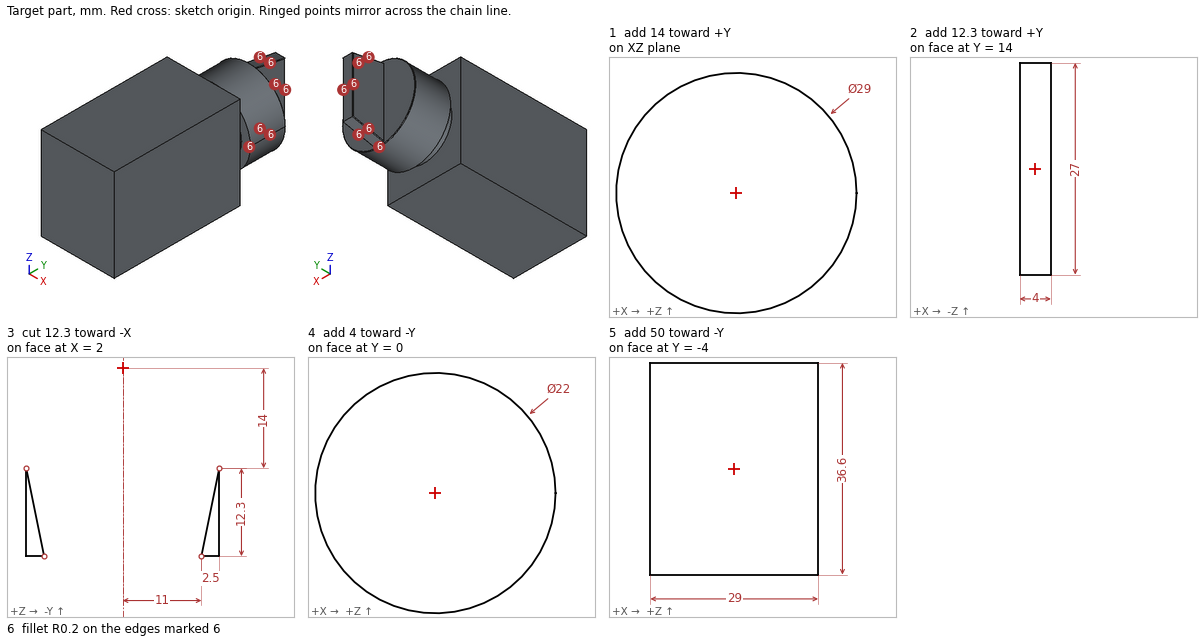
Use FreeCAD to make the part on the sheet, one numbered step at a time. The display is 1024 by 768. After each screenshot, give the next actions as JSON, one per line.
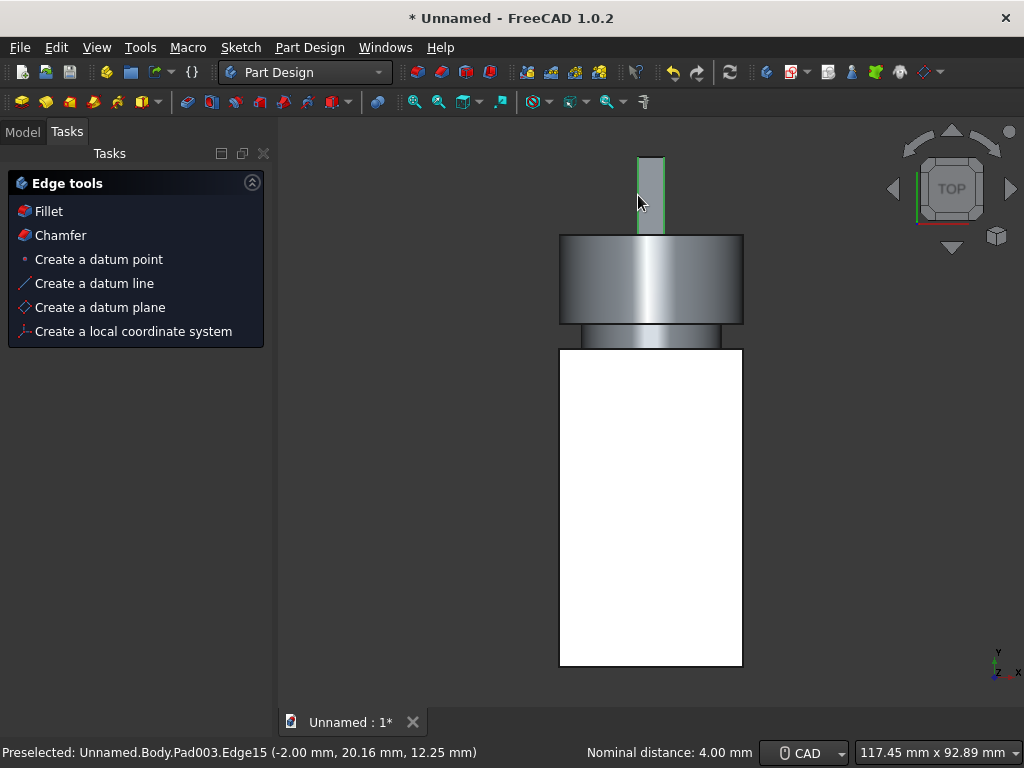
{"action": "key", "text": "0"}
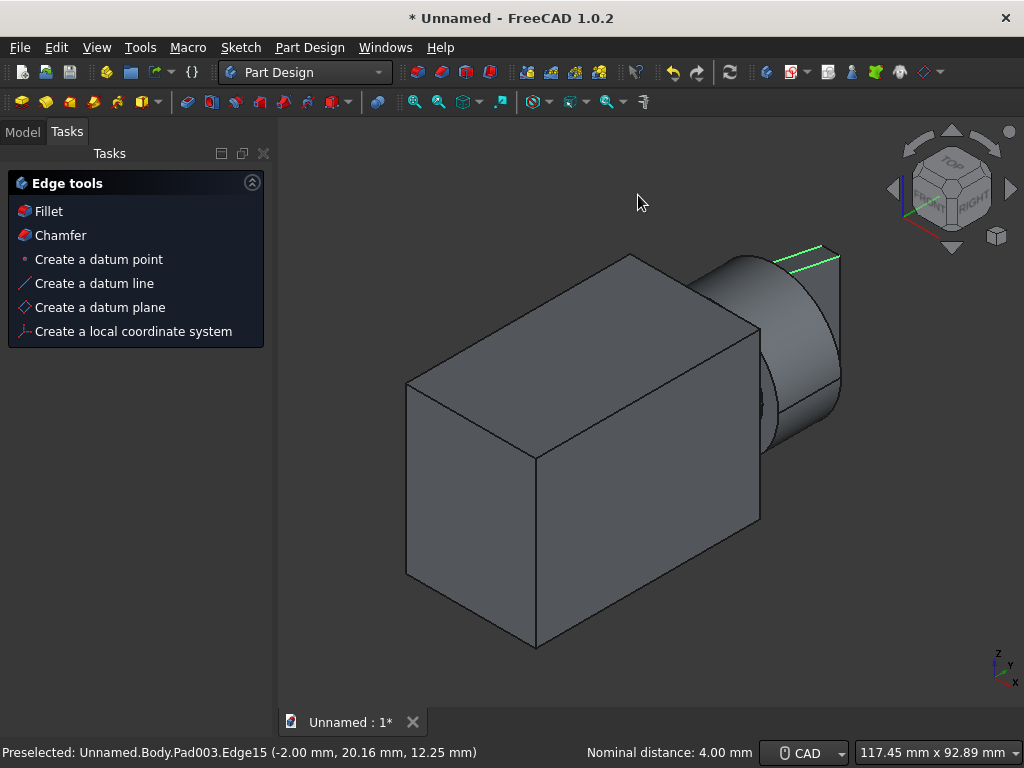
{"action": "key", "text": "1"}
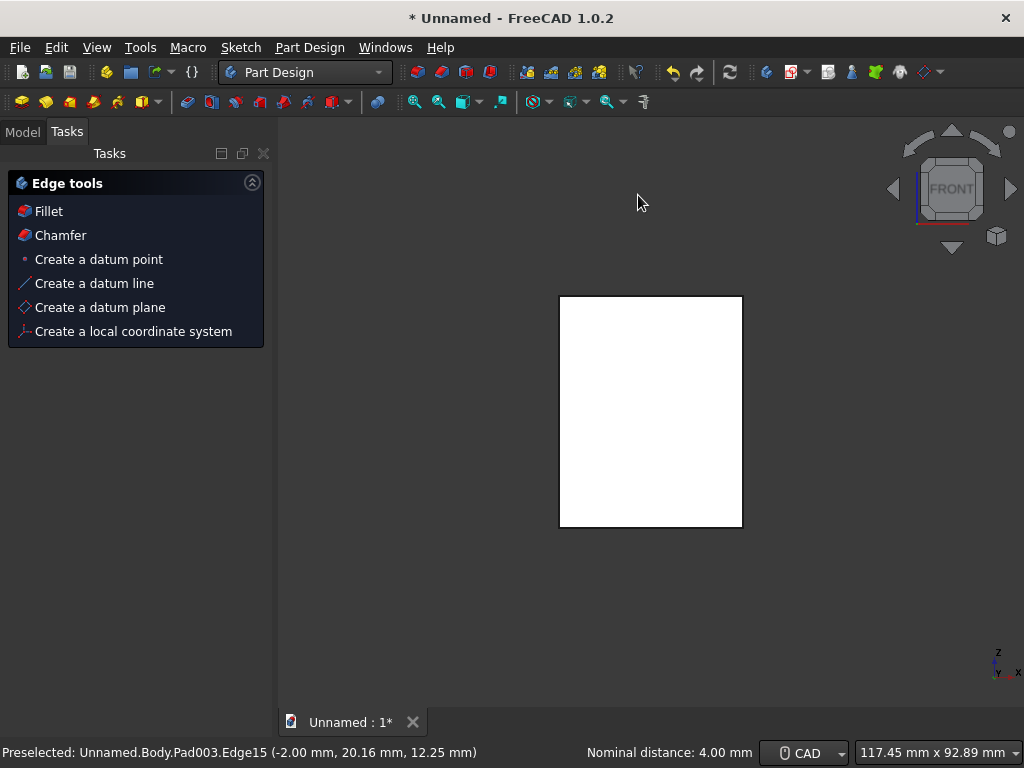
{"action": "key", "text": "v f"}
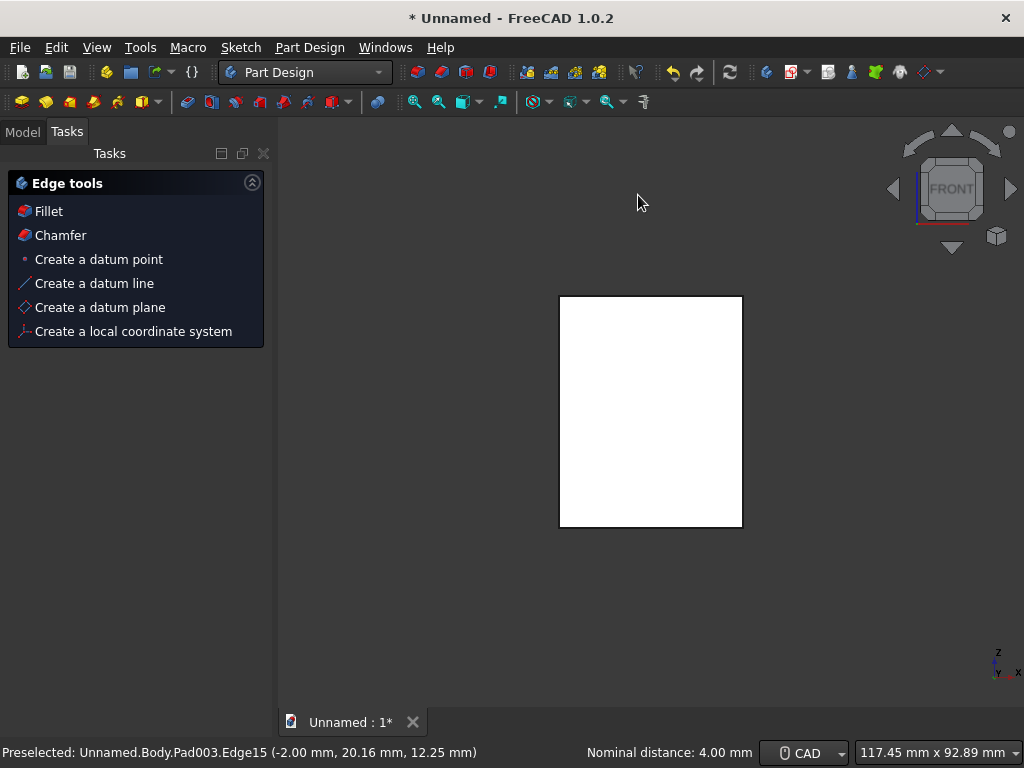
{"action": "key", "text": "3"}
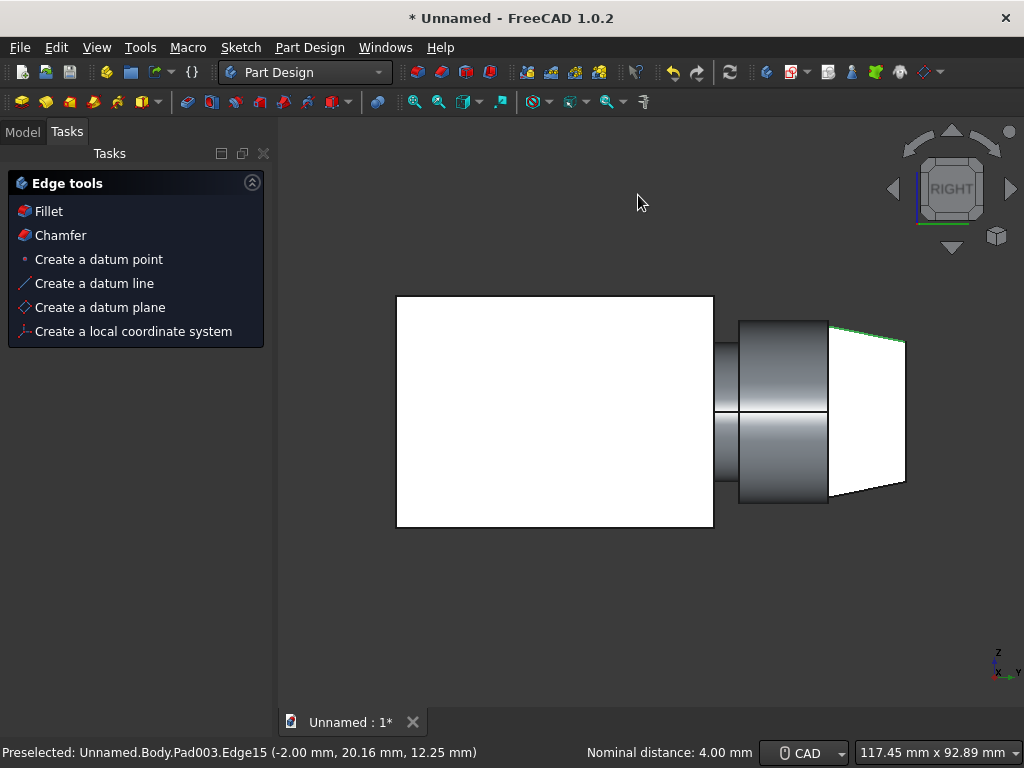
{"action": "left_click", "coordinate": [906, 411], "text": "ctrl"}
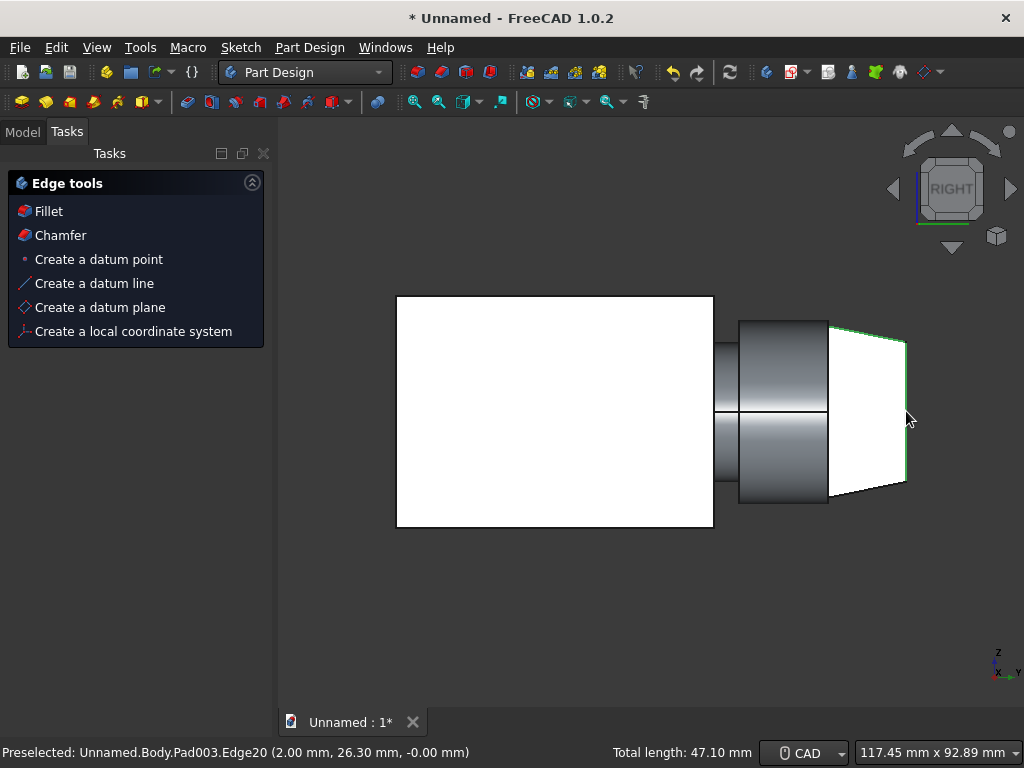
{"action": "left_click", "coordinate": [867, 489], "text": "ctrl"}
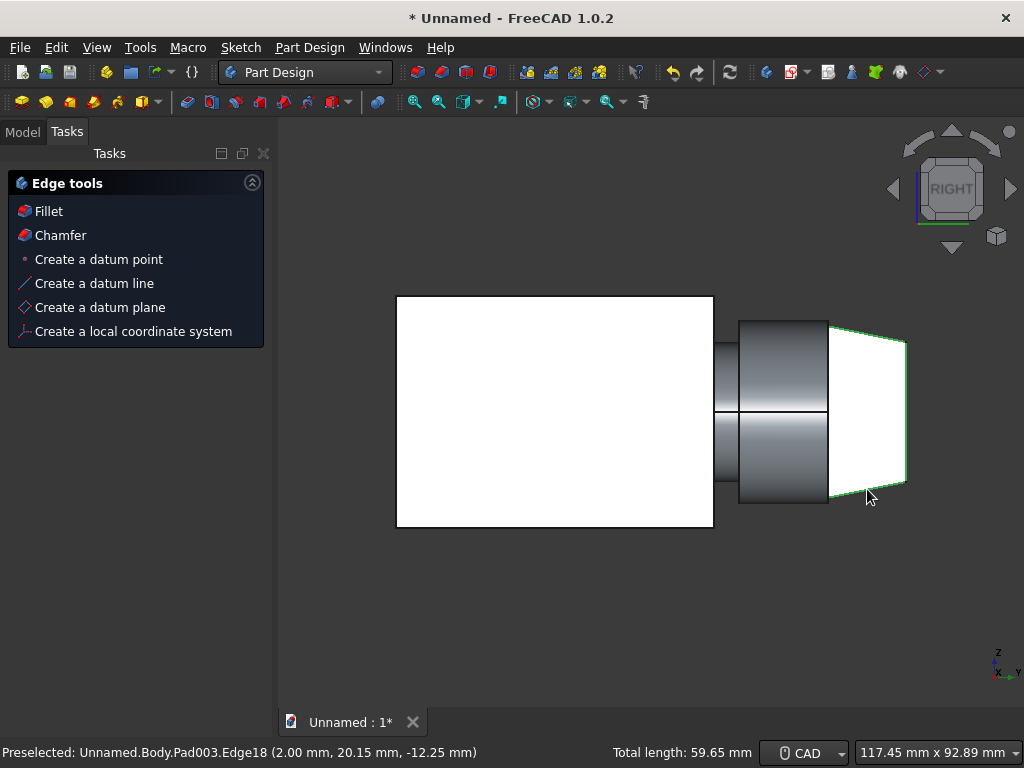
{"action": "left_click", "coordinate": [828, 502], "text": "ctrl"}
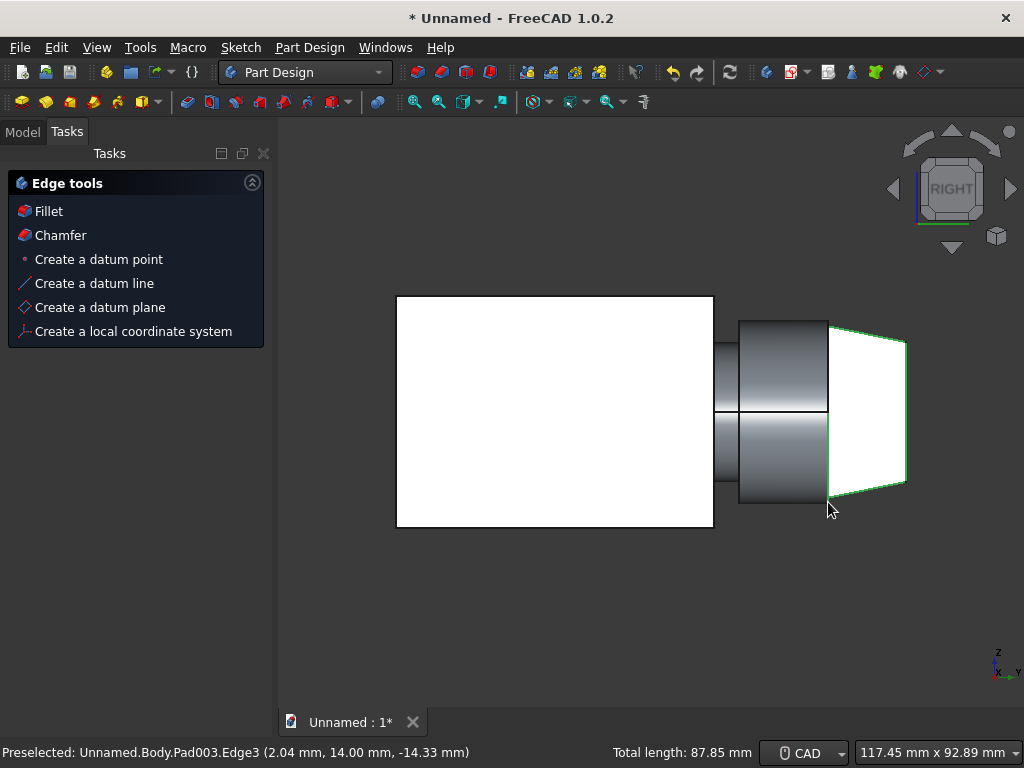
{"action": "key", "text": "5"}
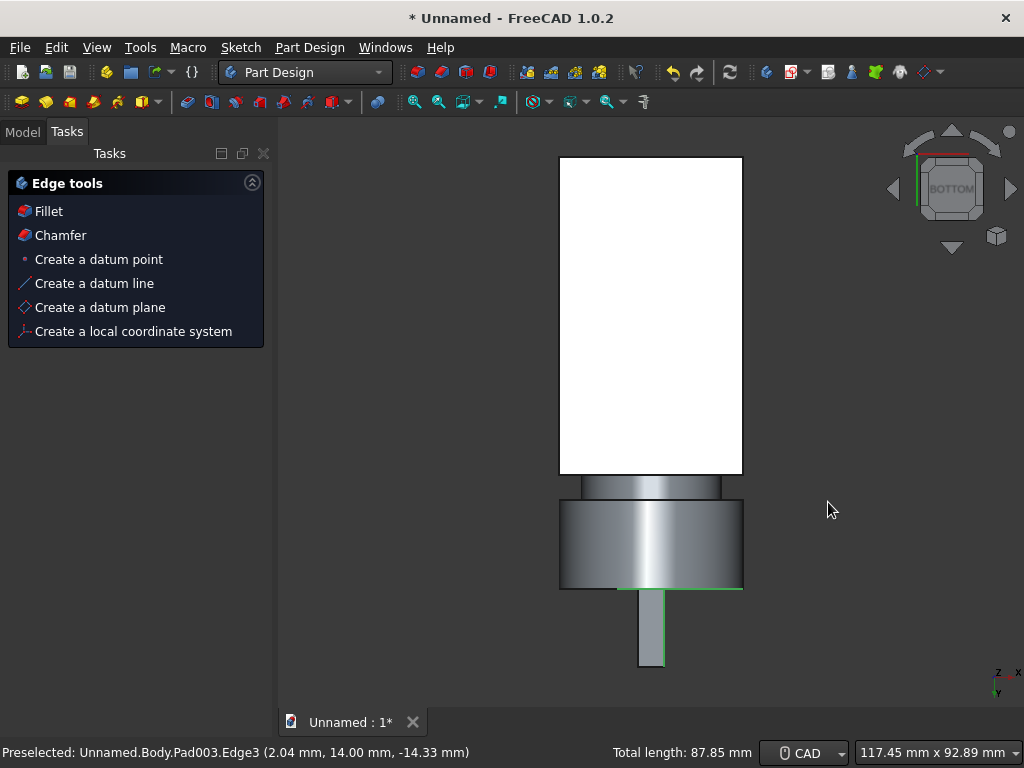
{"action": "left_click", "coordinate": [638, 627], "text": "ctrl"}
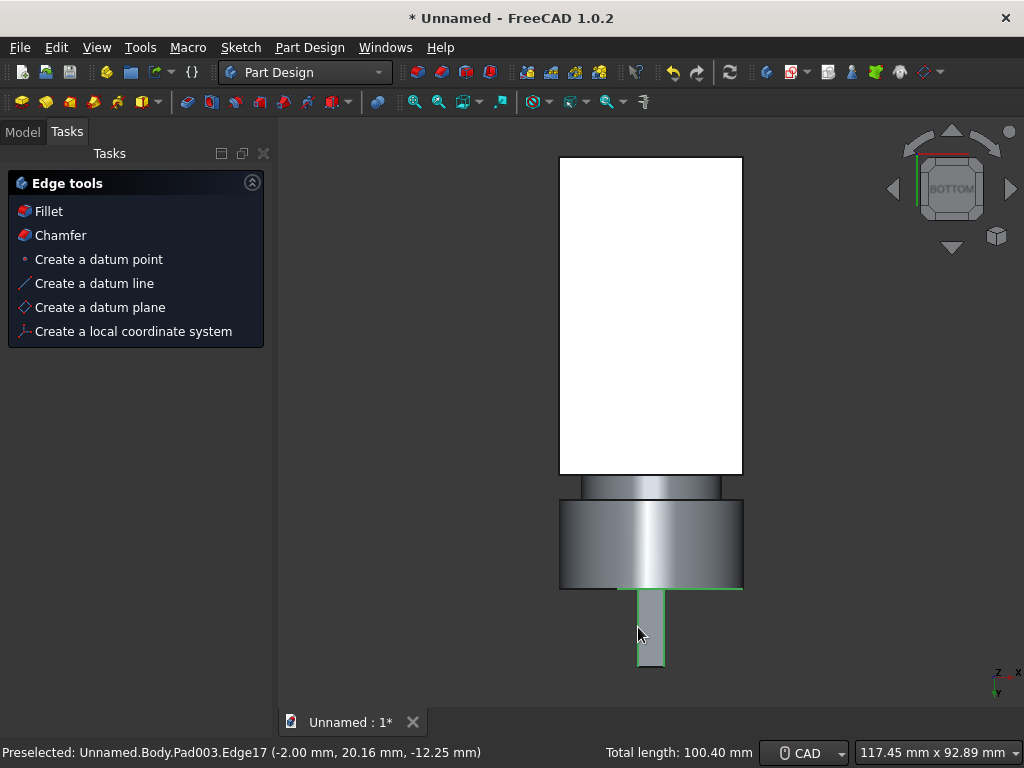
{"action": "key", "text": "4"}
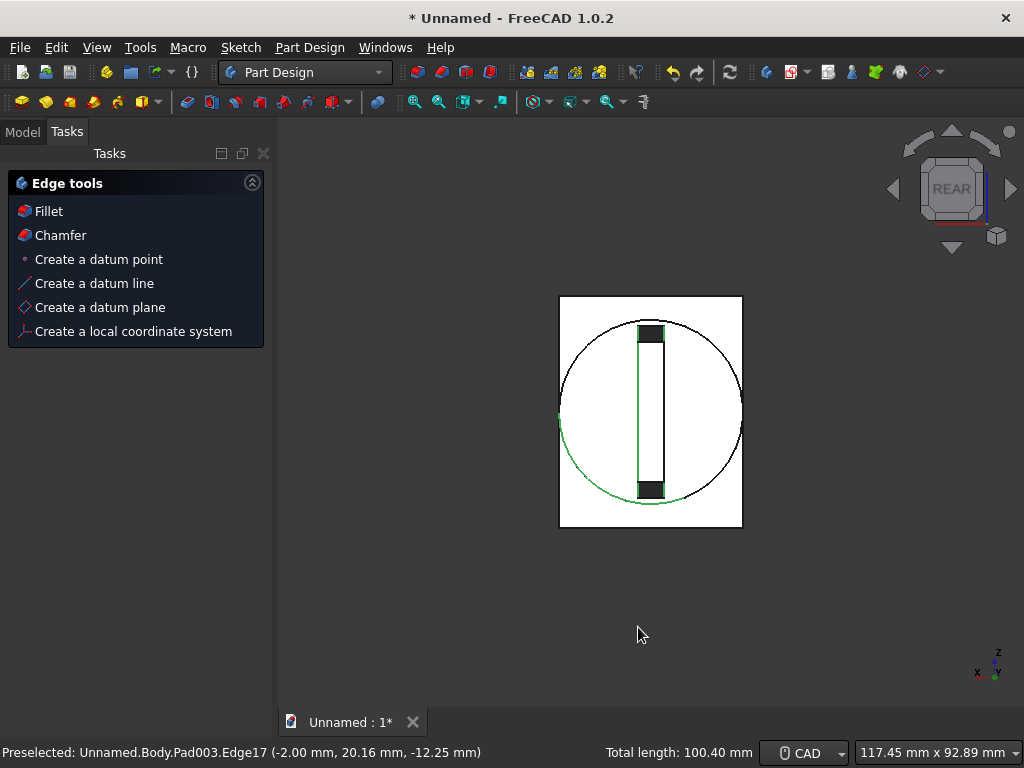
{"action": "left_click", "coordinate": [416, 102]}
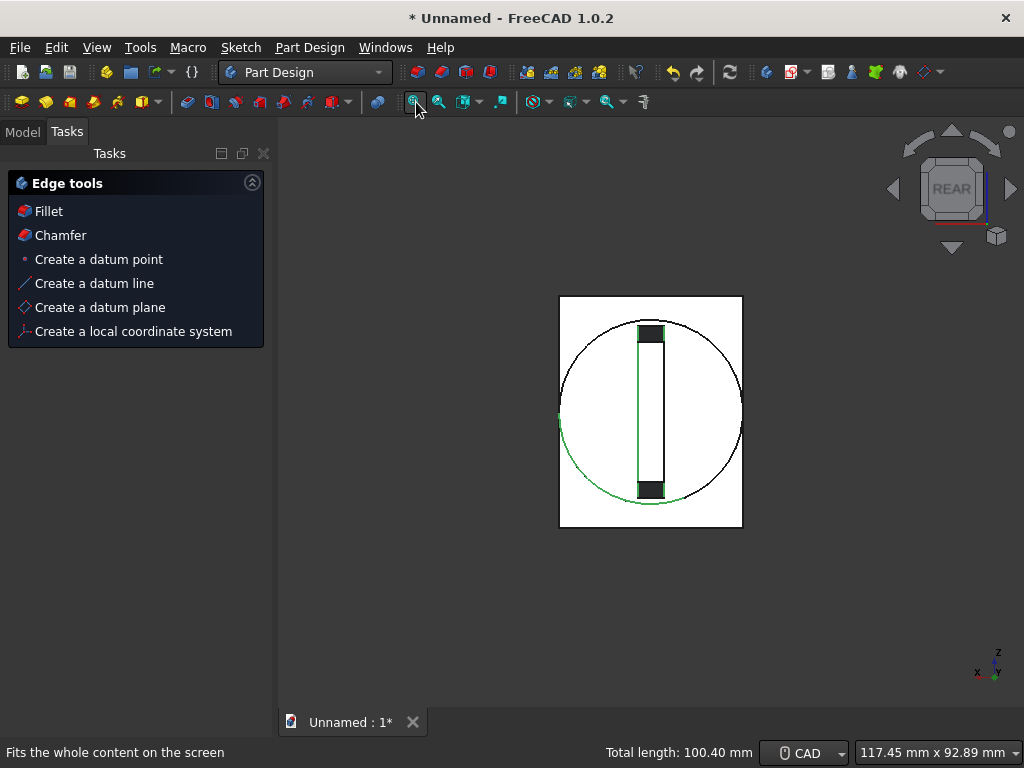
{"action": "left_click", "coordinate": [664, 411], "text": "ctrl"}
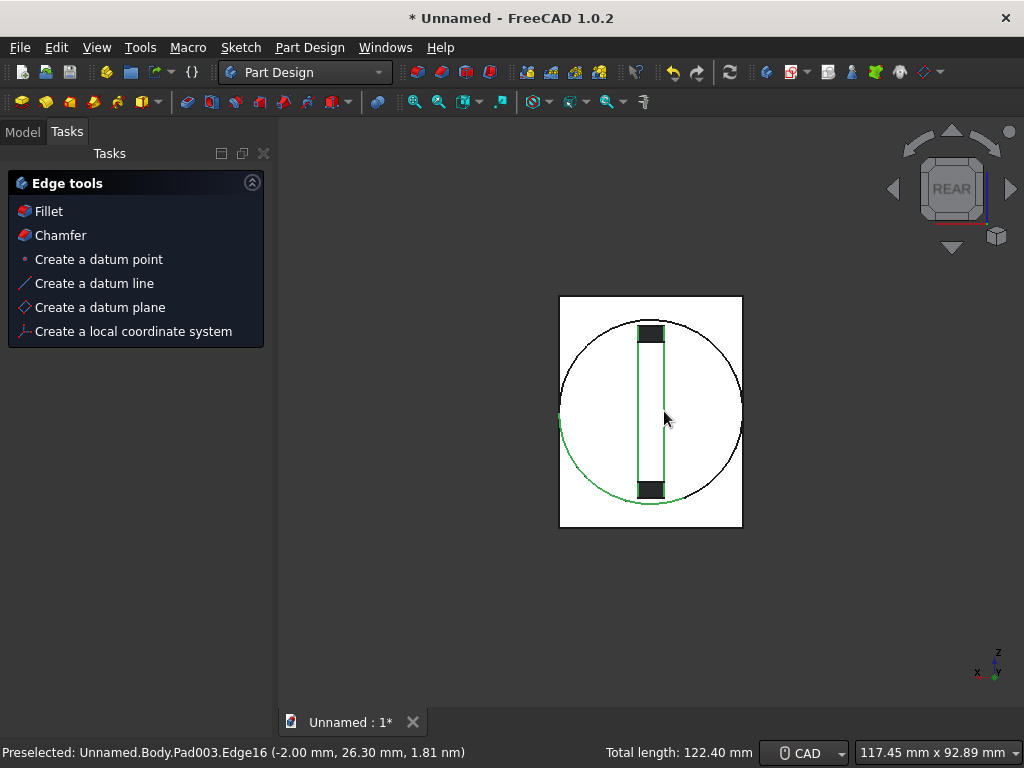
{"action": "left_click", "coordinate": [418, 72]}